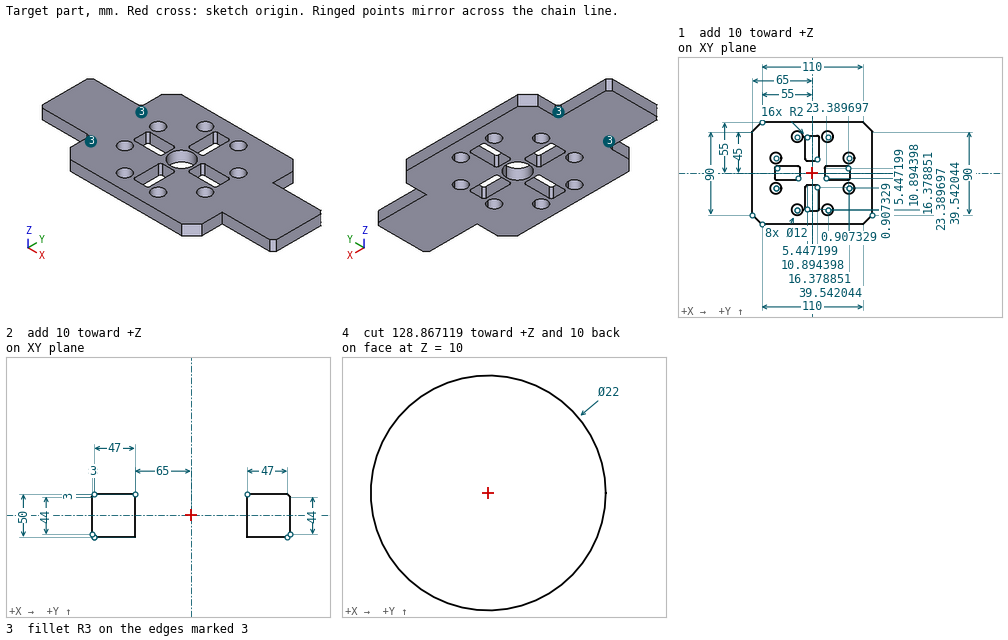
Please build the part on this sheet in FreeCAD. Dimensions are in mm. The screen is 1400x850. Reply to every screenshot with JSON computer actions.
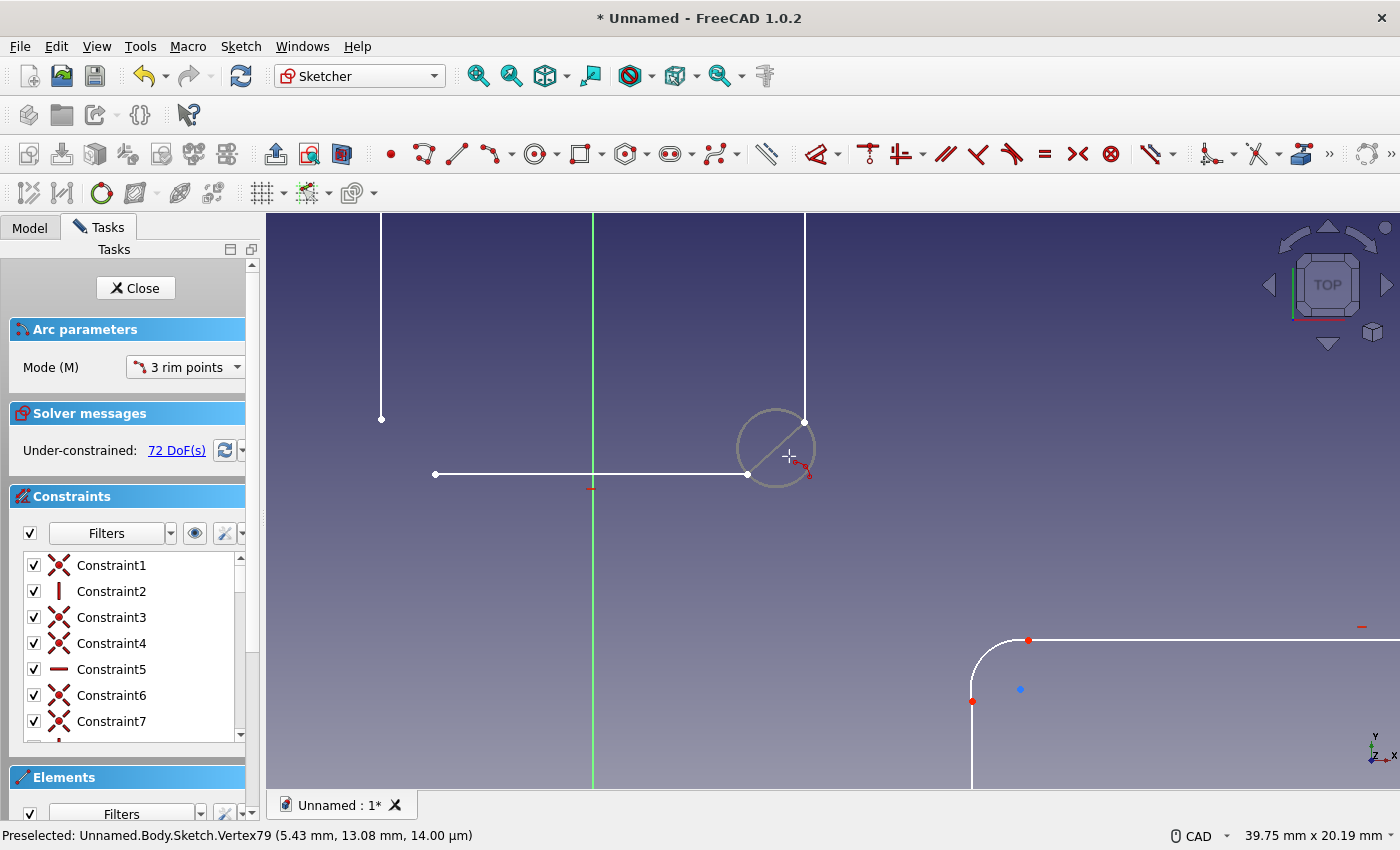
{"action": "left_click", "coordinate": [788, 453]}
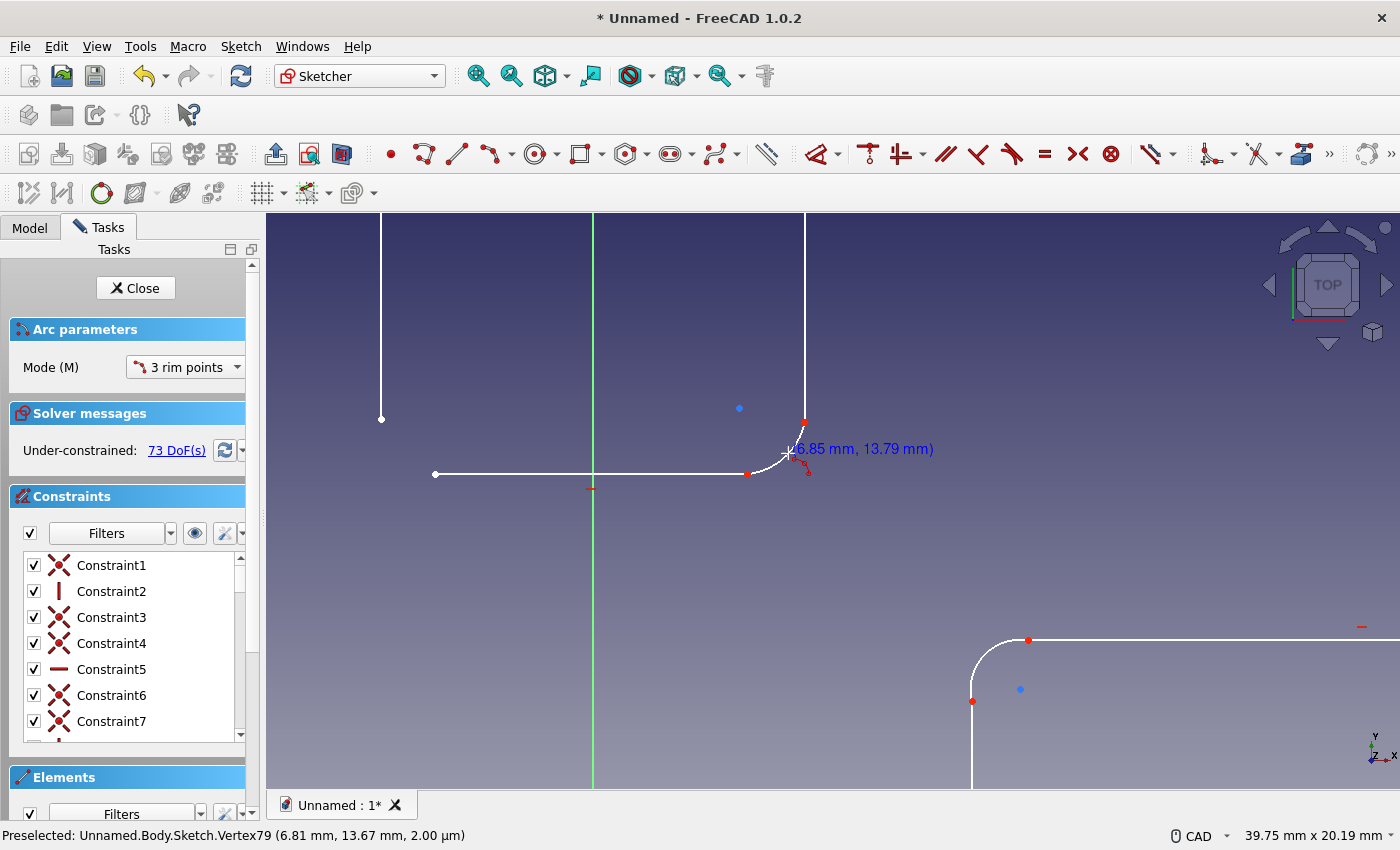
{"action": "scroll", "coordinate": [786, 458], "scroll_direction": "down", "scroll_amount": 11}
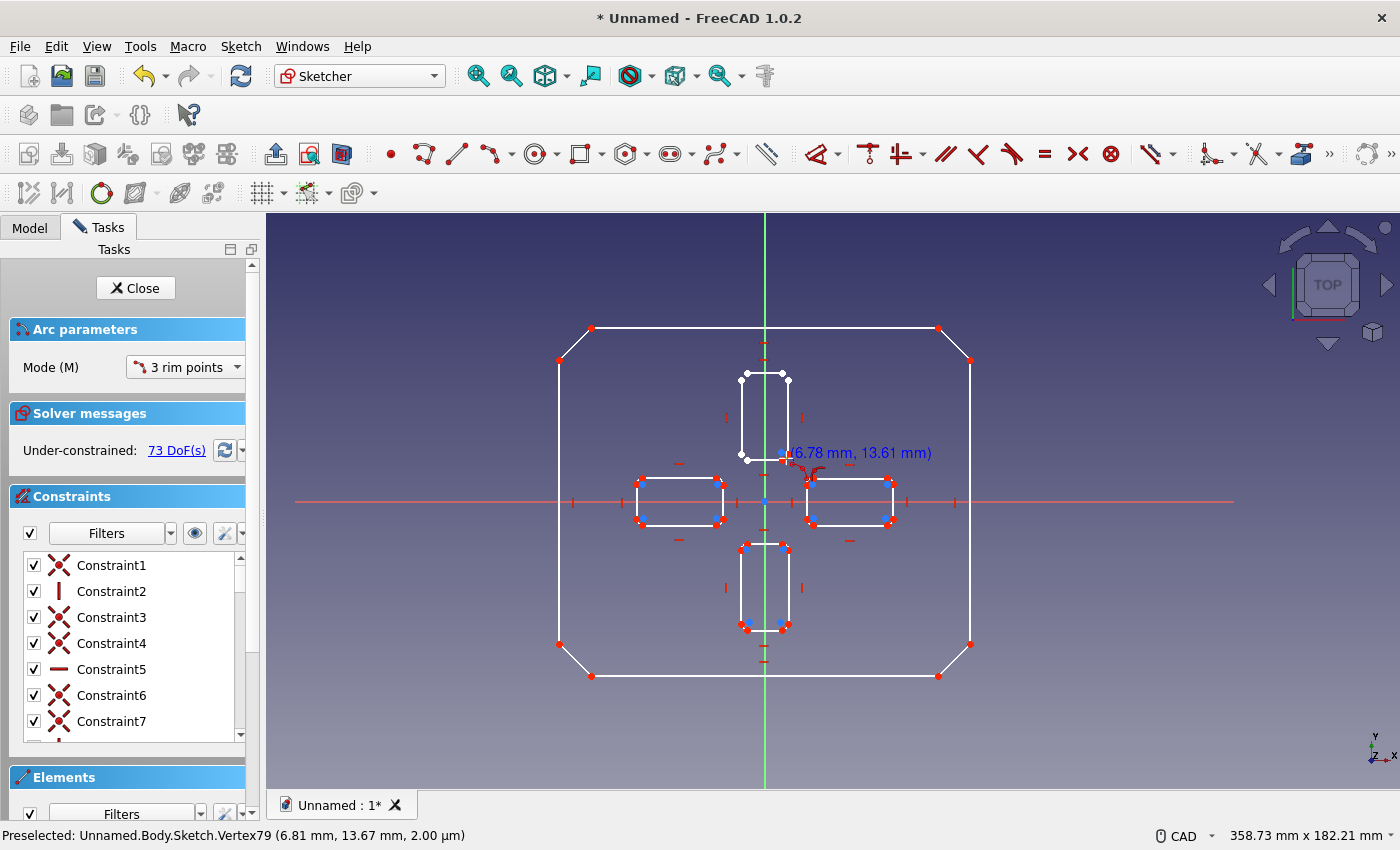
{"action": "scroll", "coordinate": [748, 460], "scroll_direction": "up", "scroll_amount": 3}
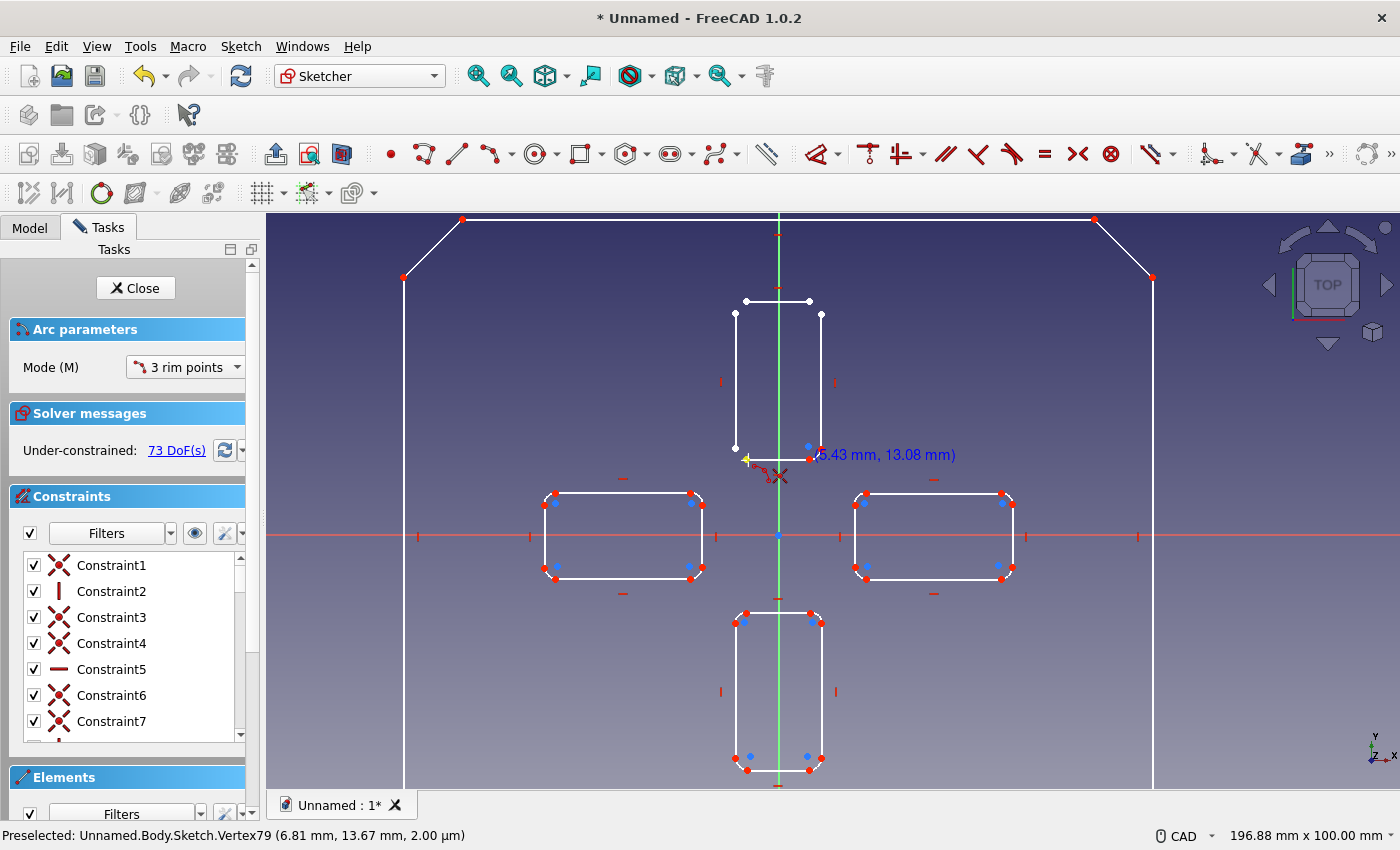
{"action": "left_click", "coordinate": [747, 460]}
{"action": "left_click", "coordinate": [736, 449]}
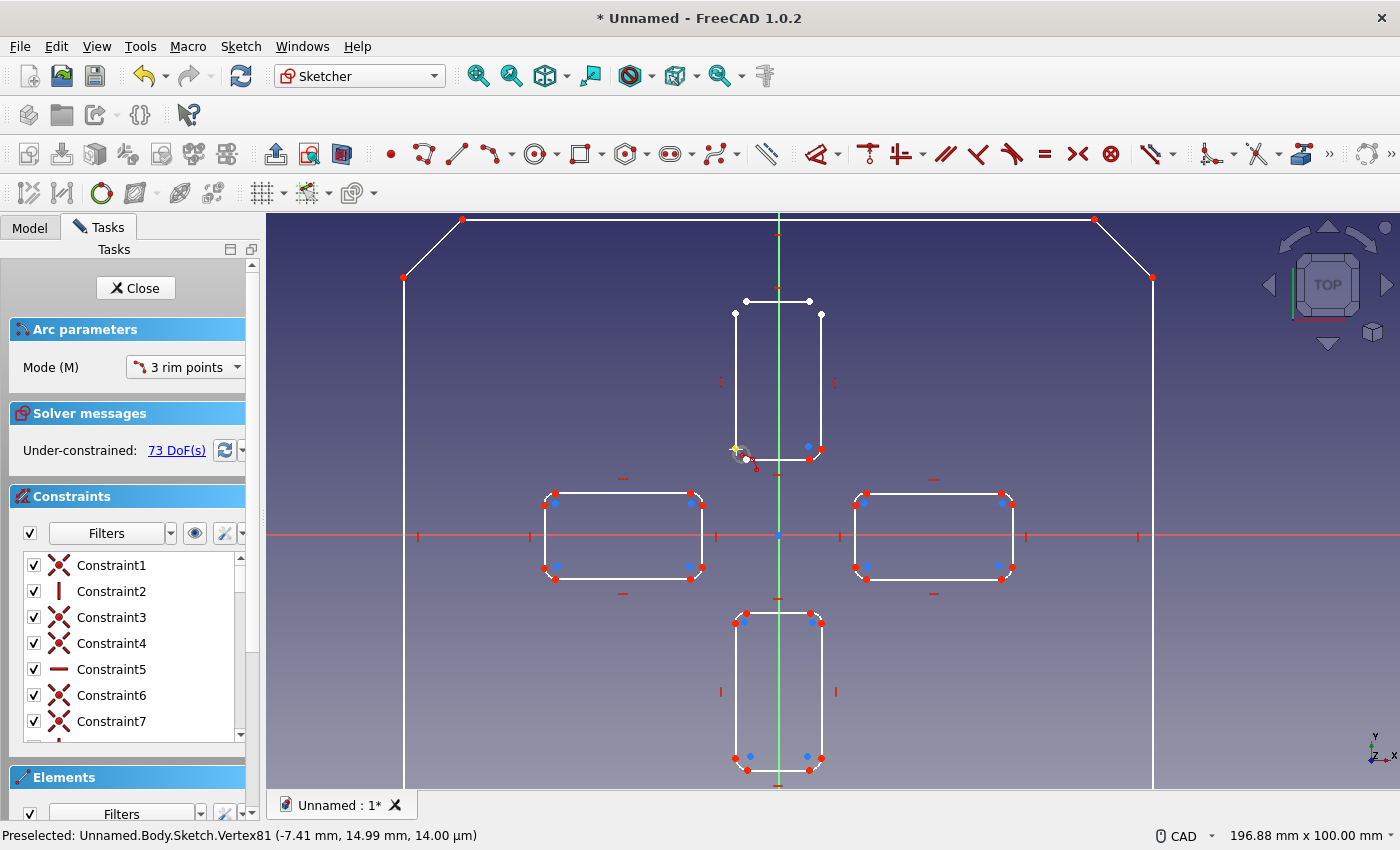
{"action": "scroll", "coordinate": [739, 456], "scroll_direction": "up", "scroll_amount": 8}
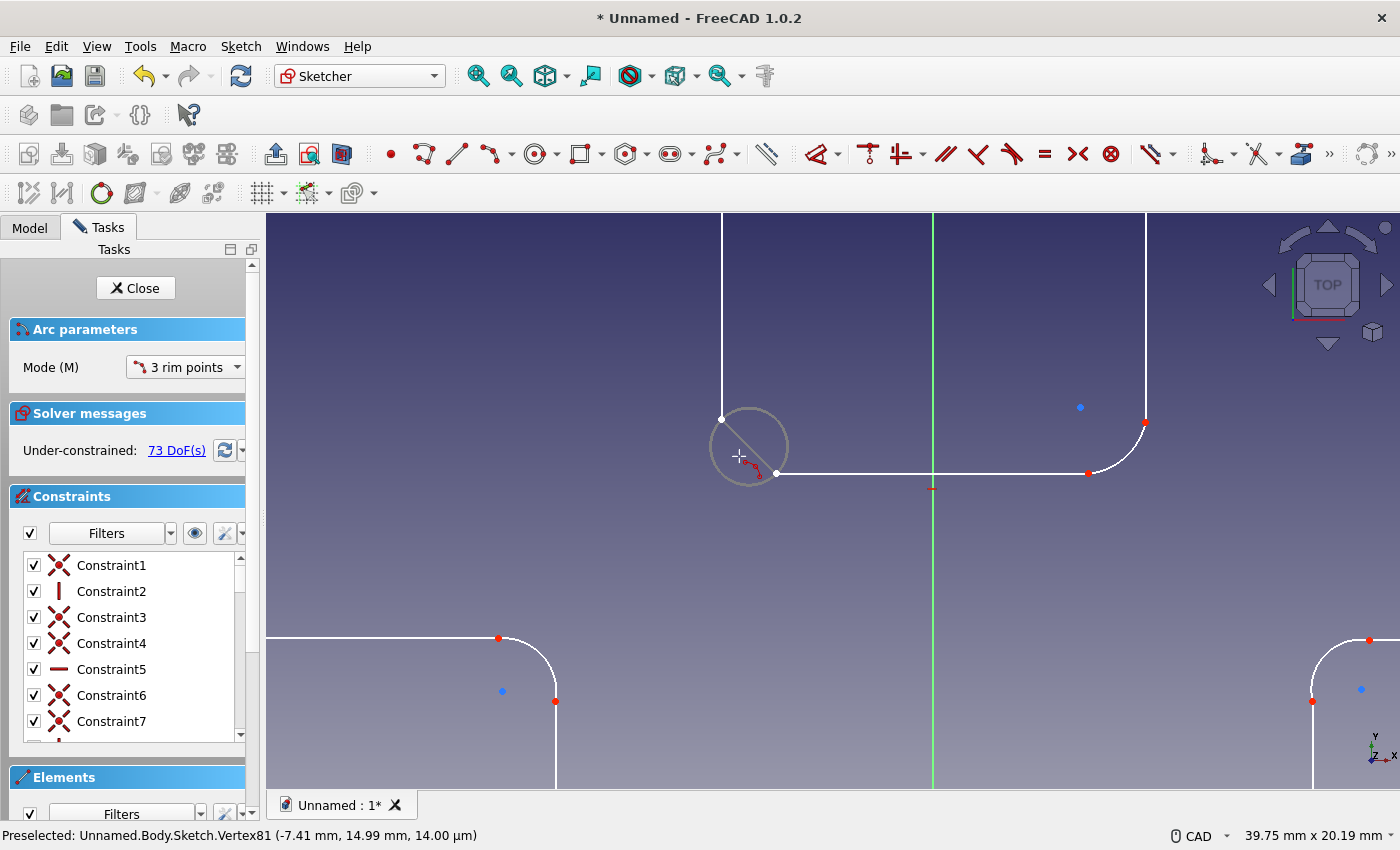
{"action": "left_click", "coordinate": [738, 453]}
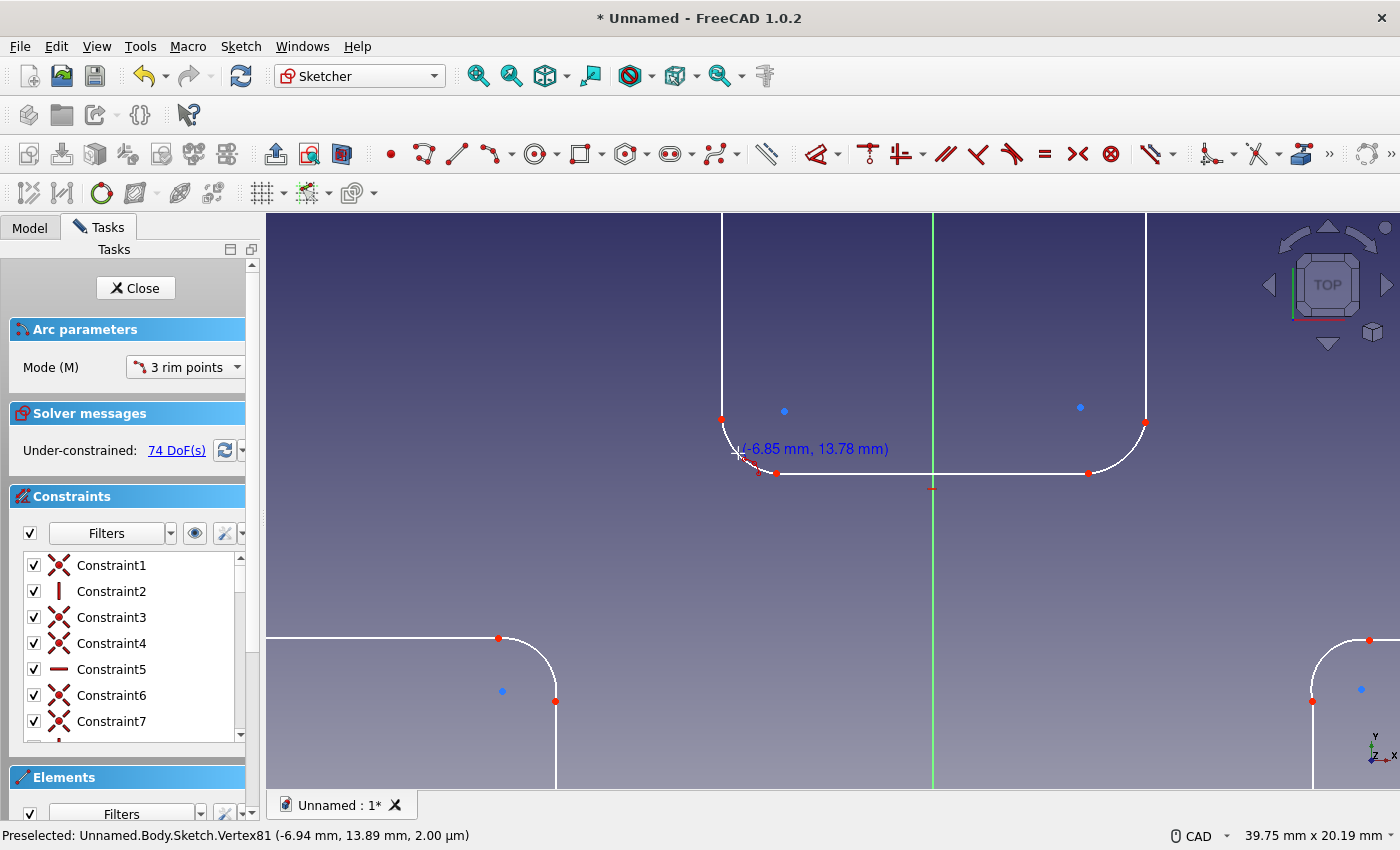
{"action": "scroll", "coordinate": [743, 458], "scroll_direction": "down", "scroll_amount": 11}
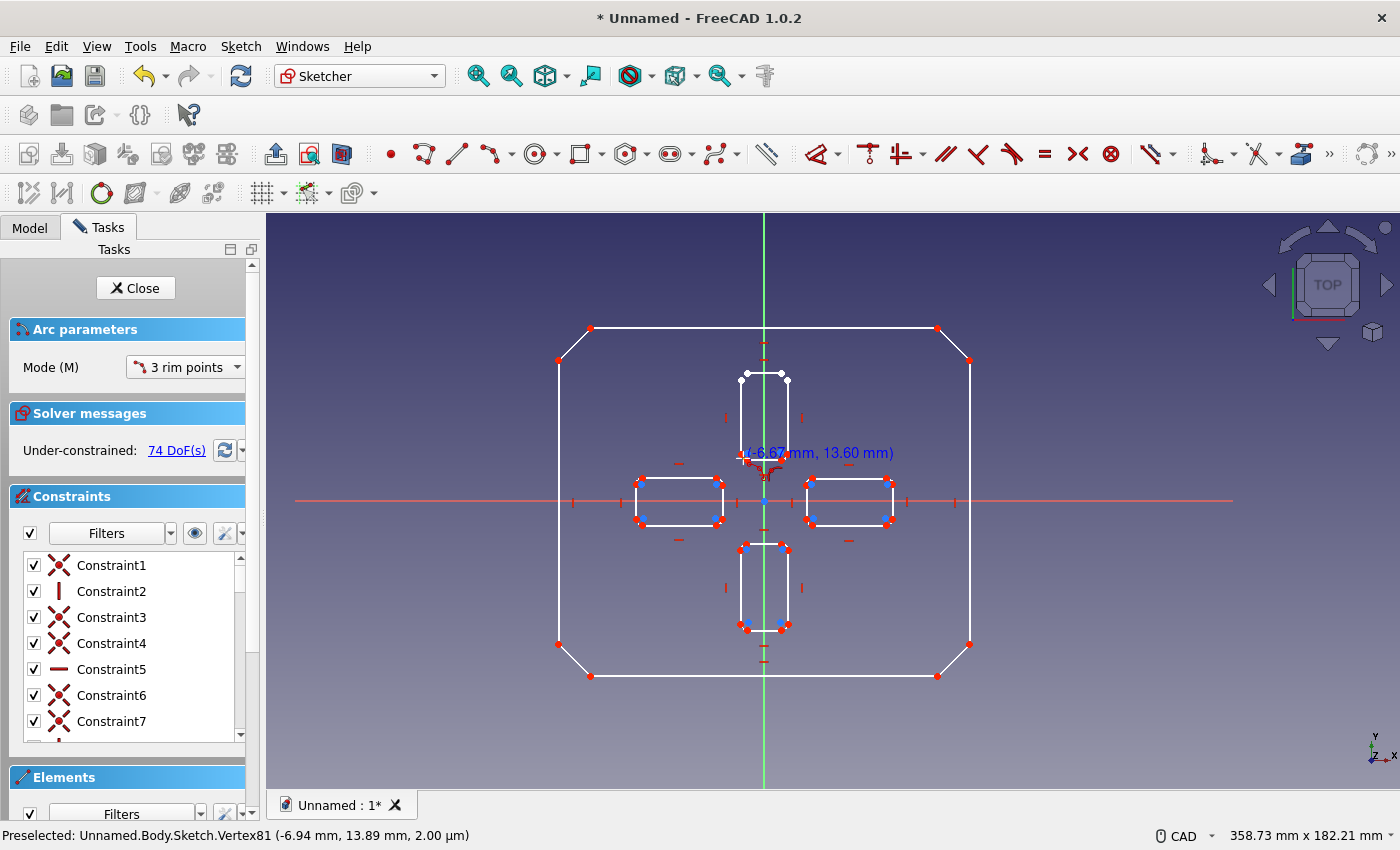
{"action": "scroll", "coordinate": [741, 379], "scroll_direction": "up", "scroll_amount": 3}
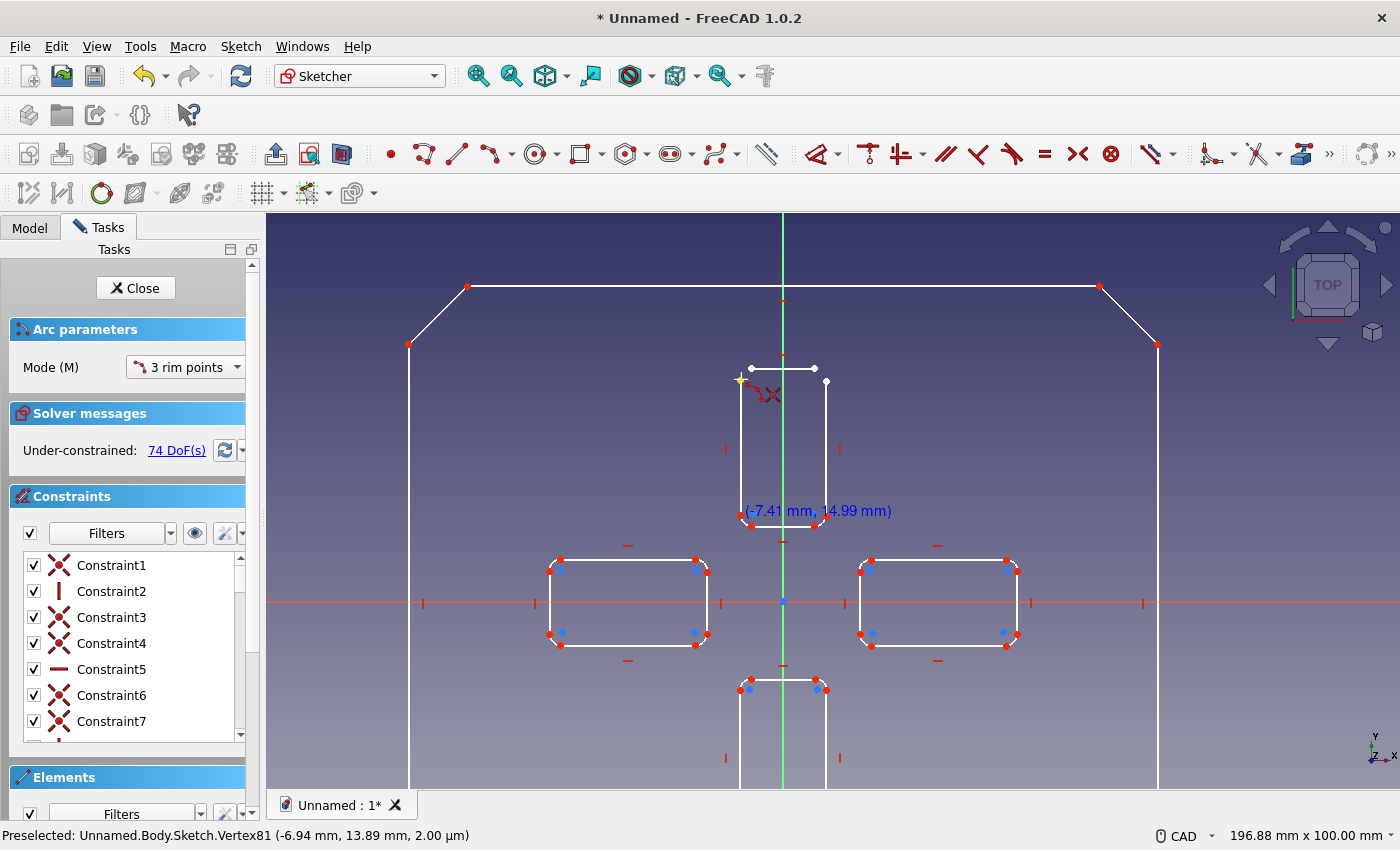
{"action": "left_click", "coordinate": [741, 381]}
{"action": "left_click", "coordinate": [752, 369]}